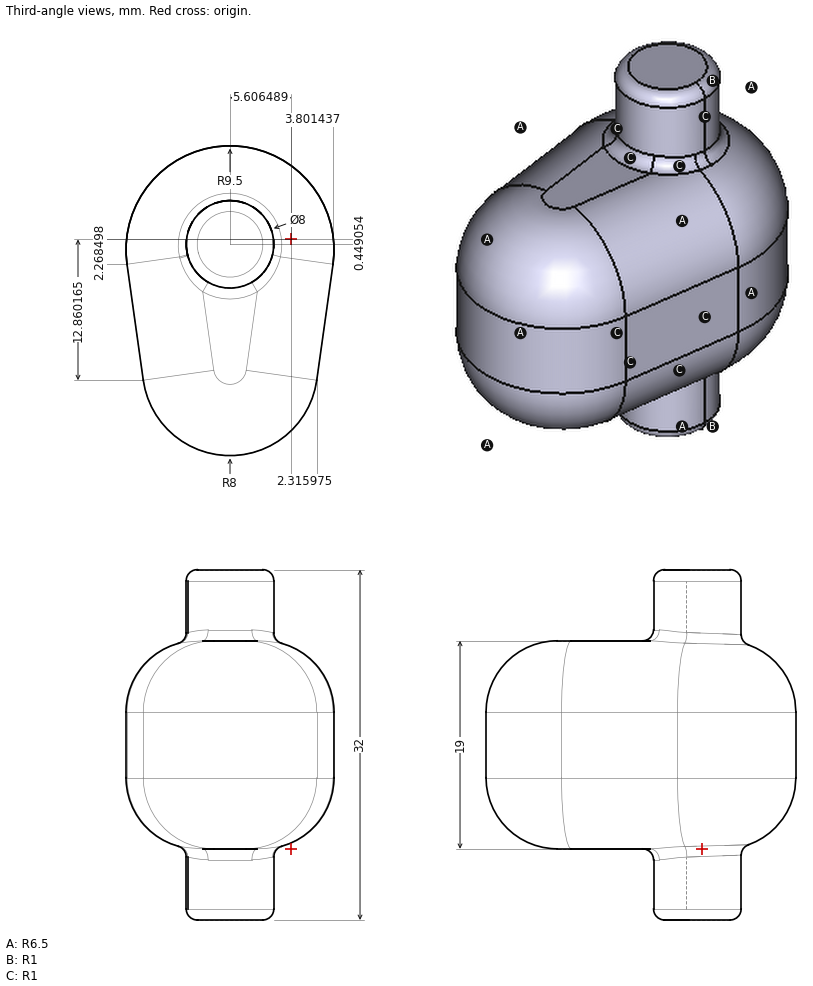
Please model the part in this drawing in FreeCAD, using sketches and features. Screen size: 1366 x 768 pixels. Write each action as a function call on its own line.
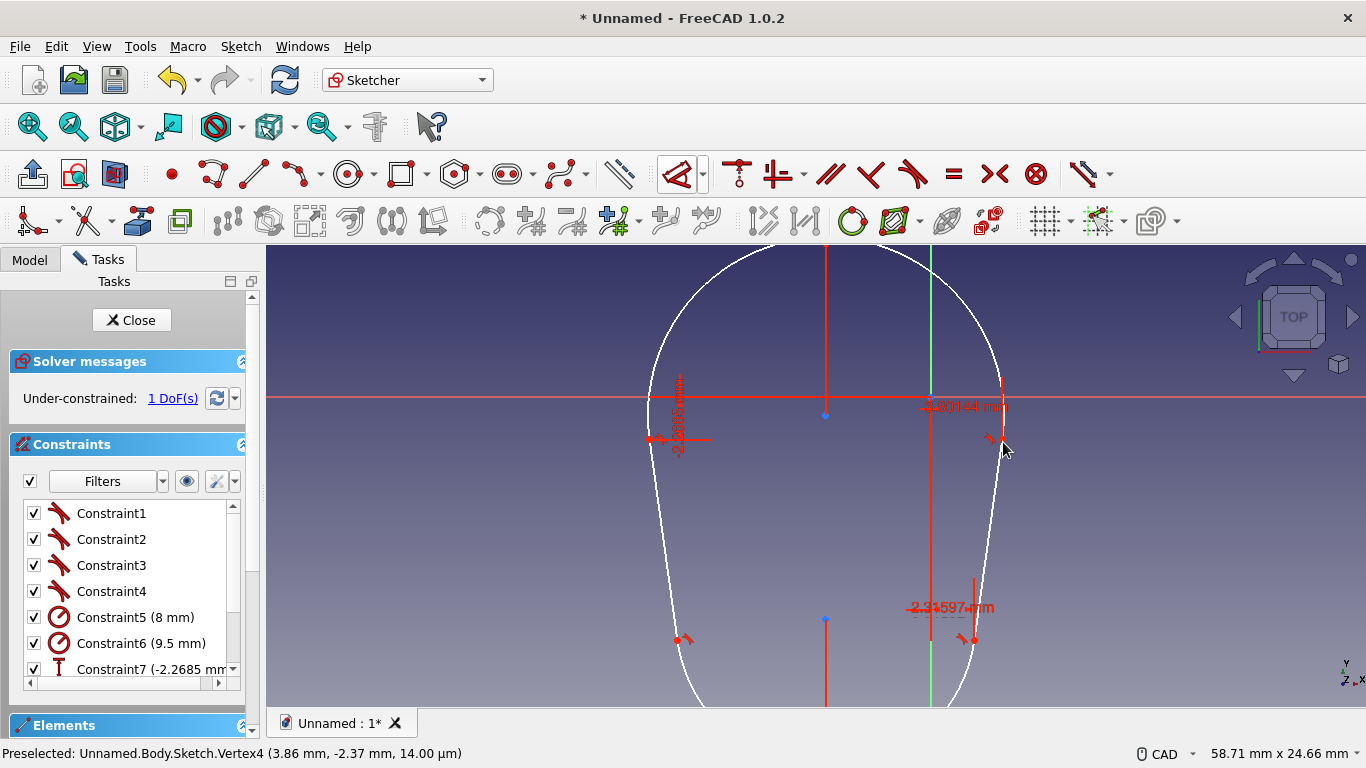
click(677, 640)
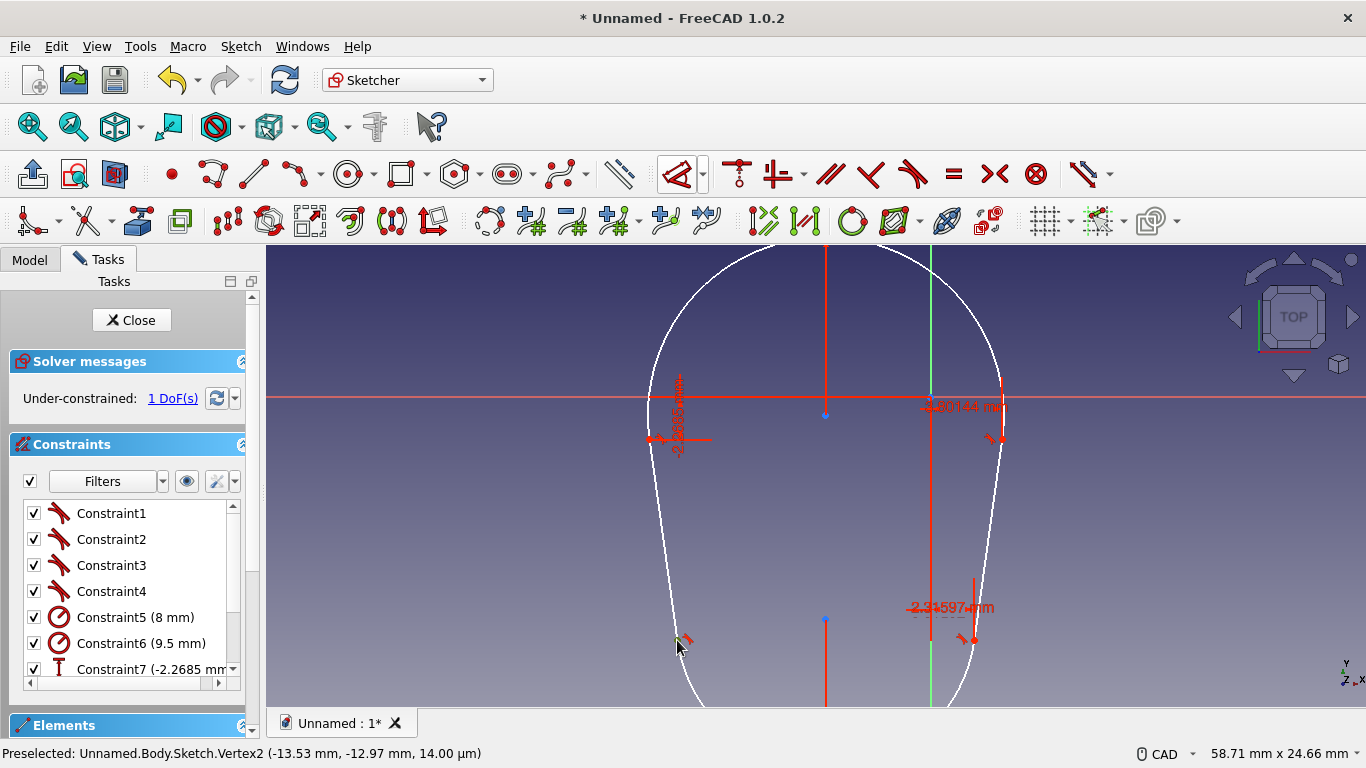
key(i)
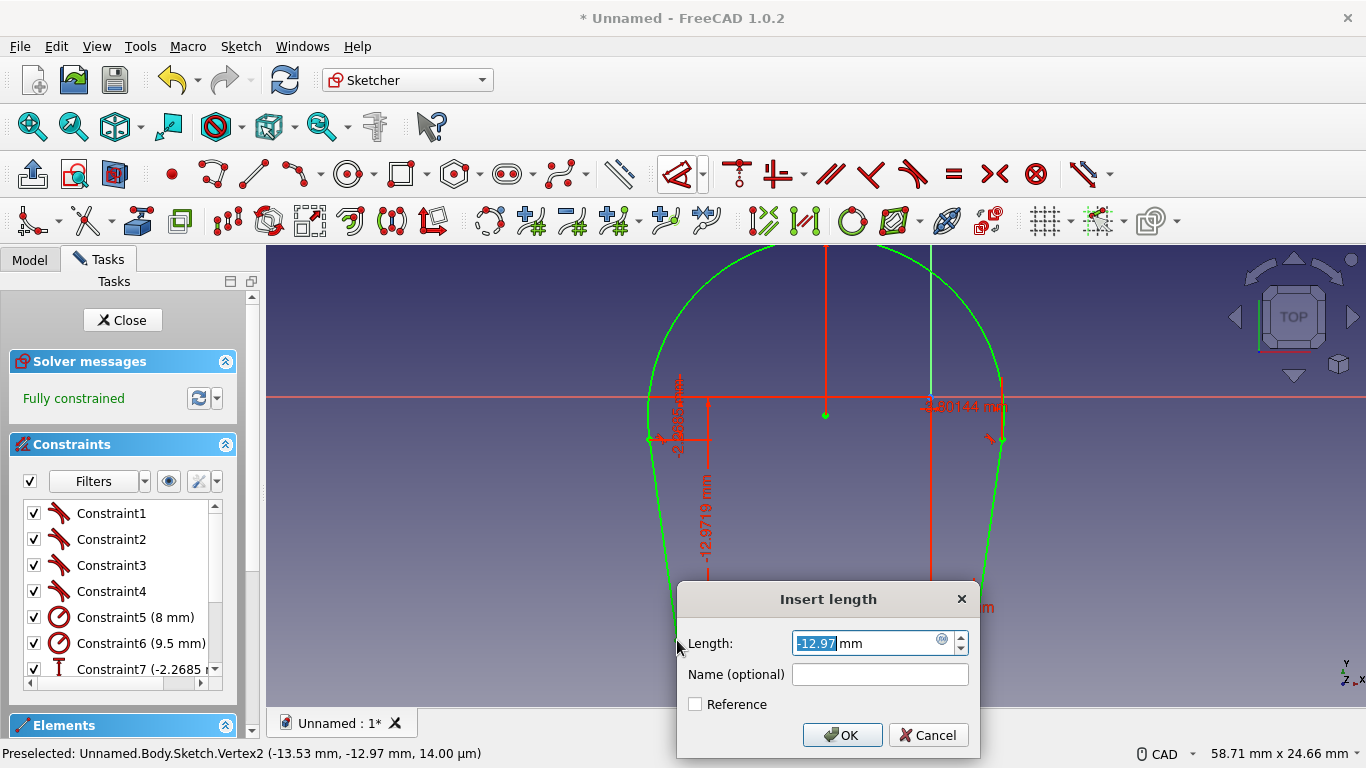
text(-12.860165)
key(Return)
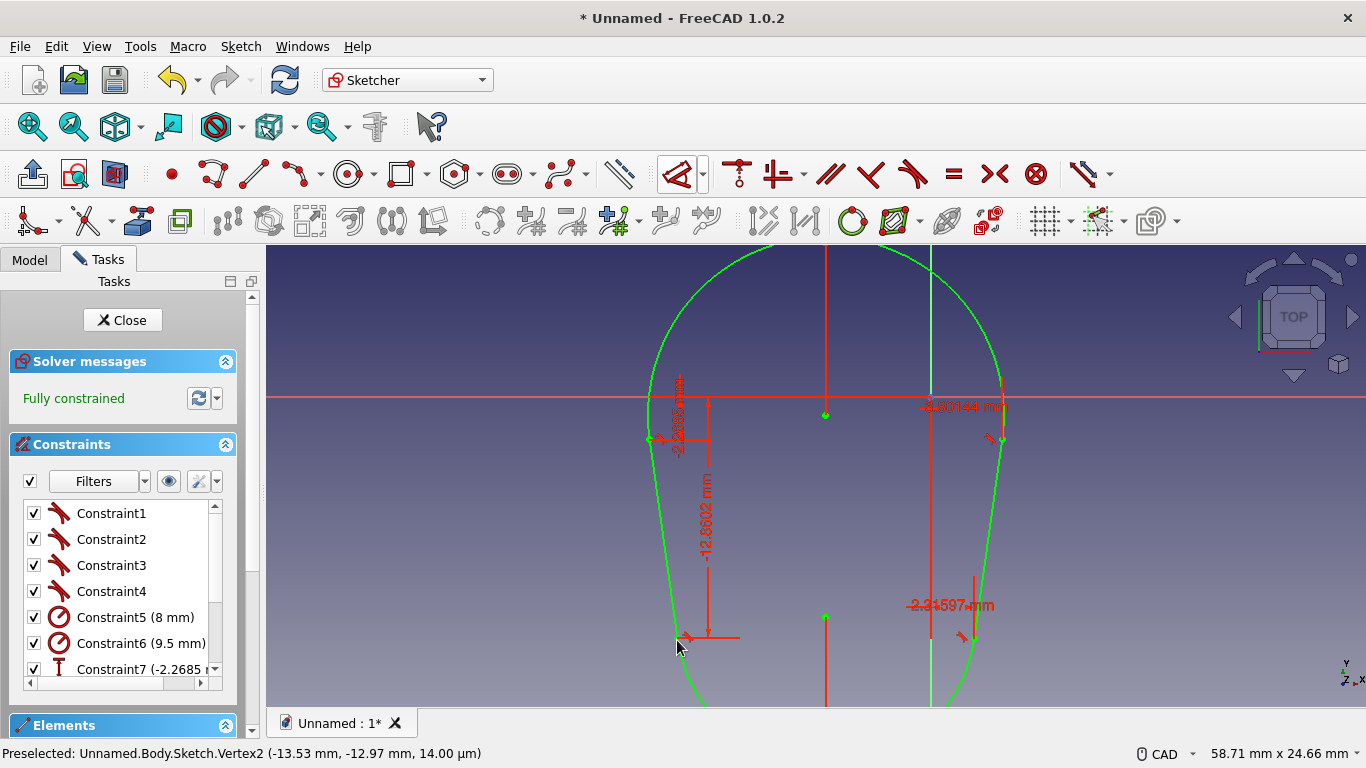
click(123, 320)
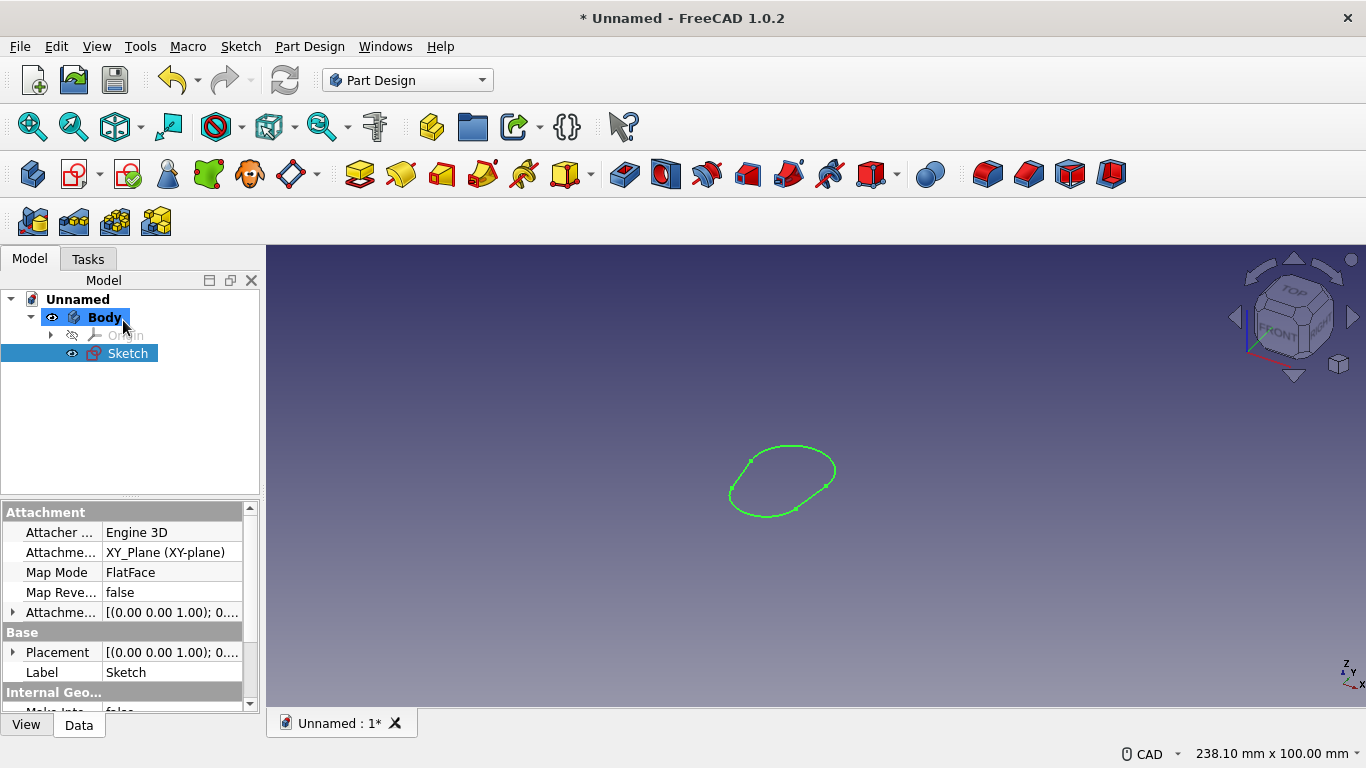
click(360, 174)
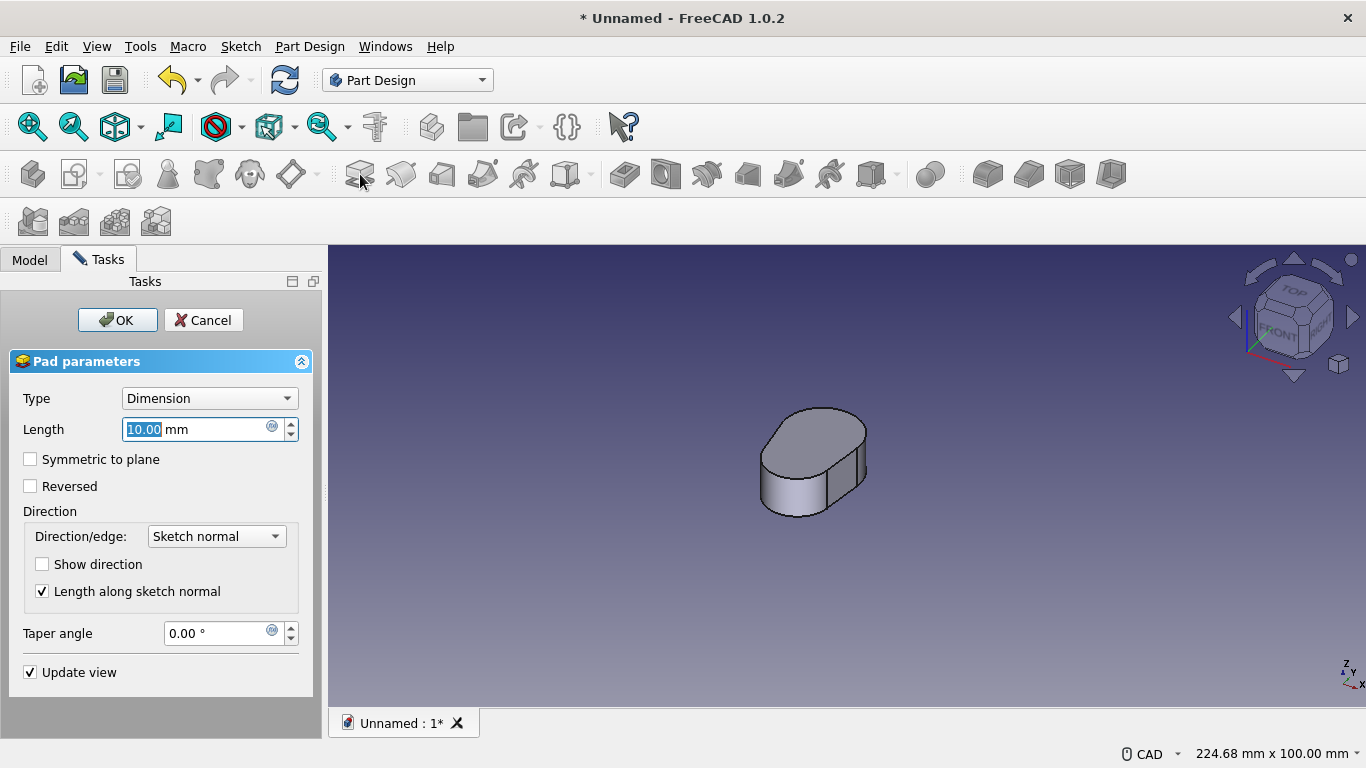
text(19)
key(Tab)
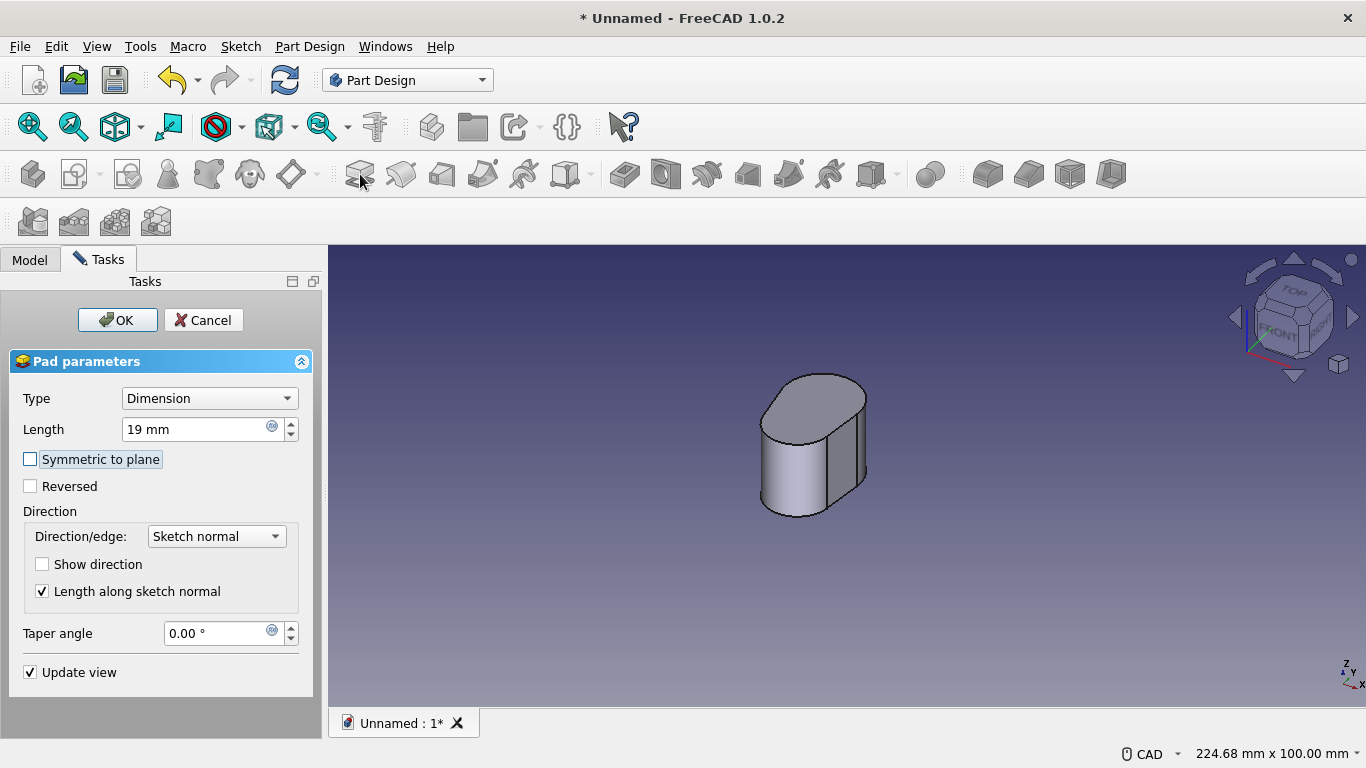
click(118, 320)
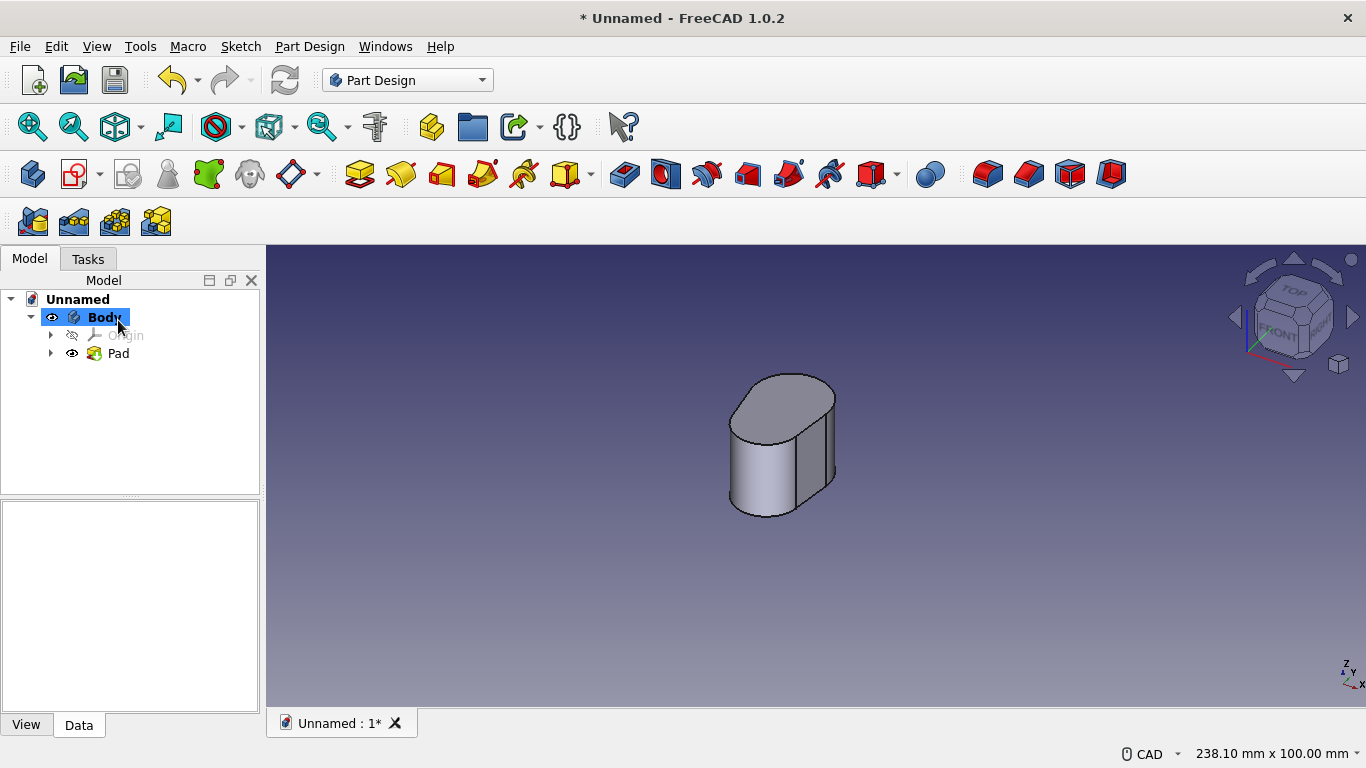
click(33, 128)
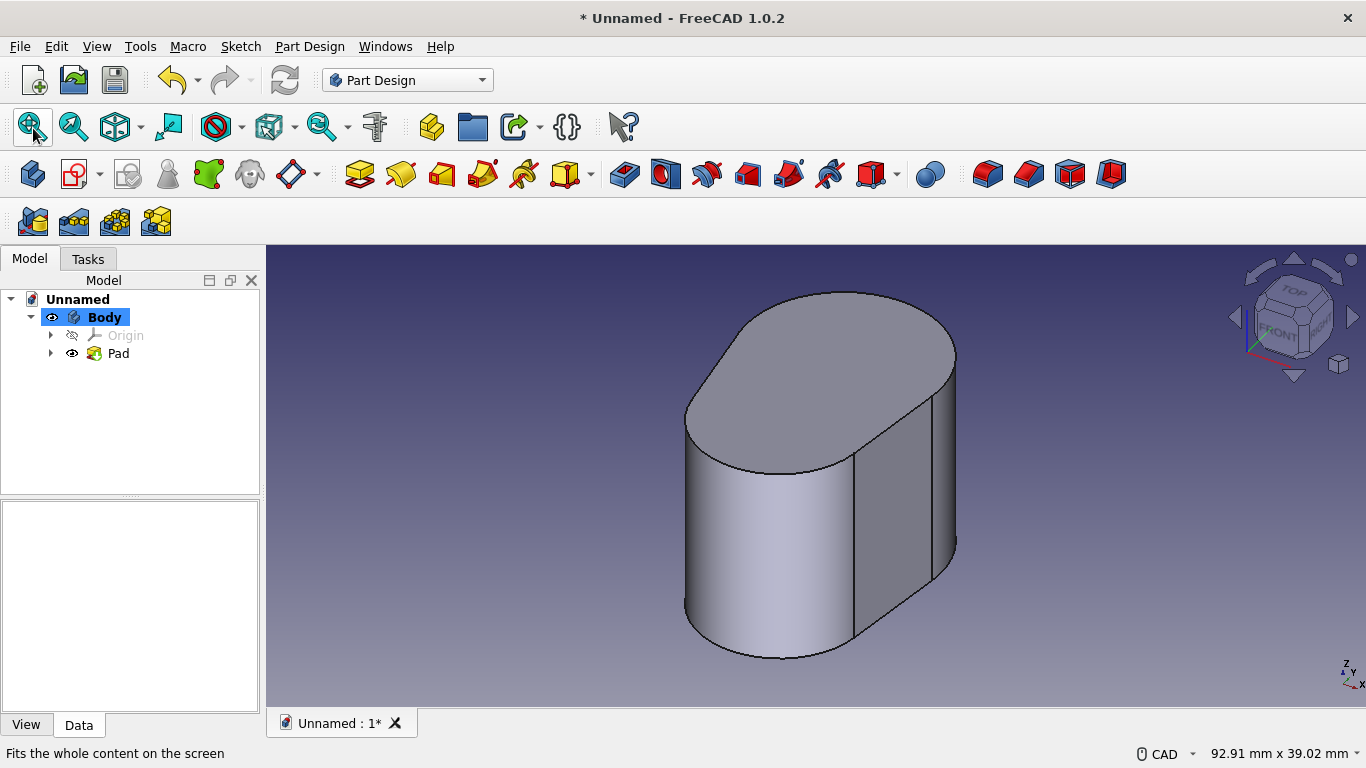
click(840, 359)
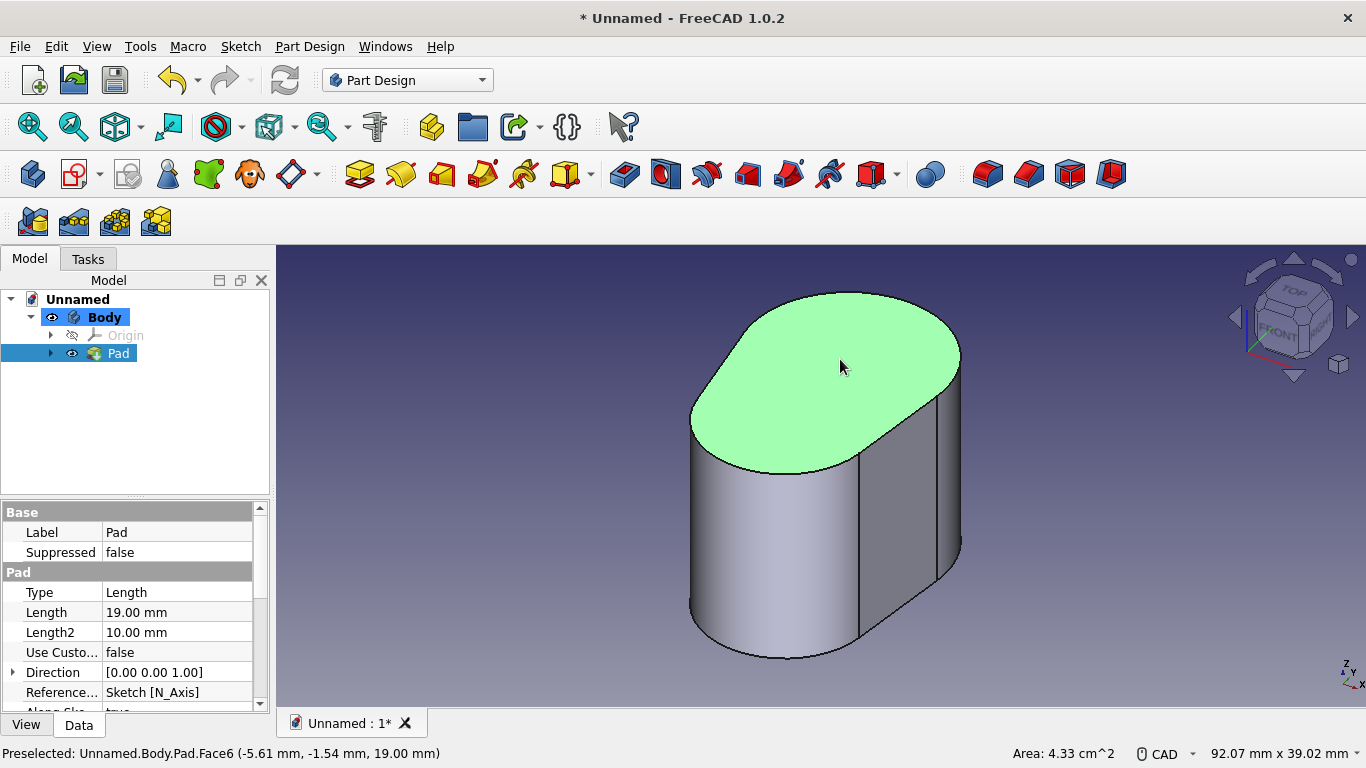
key(0)